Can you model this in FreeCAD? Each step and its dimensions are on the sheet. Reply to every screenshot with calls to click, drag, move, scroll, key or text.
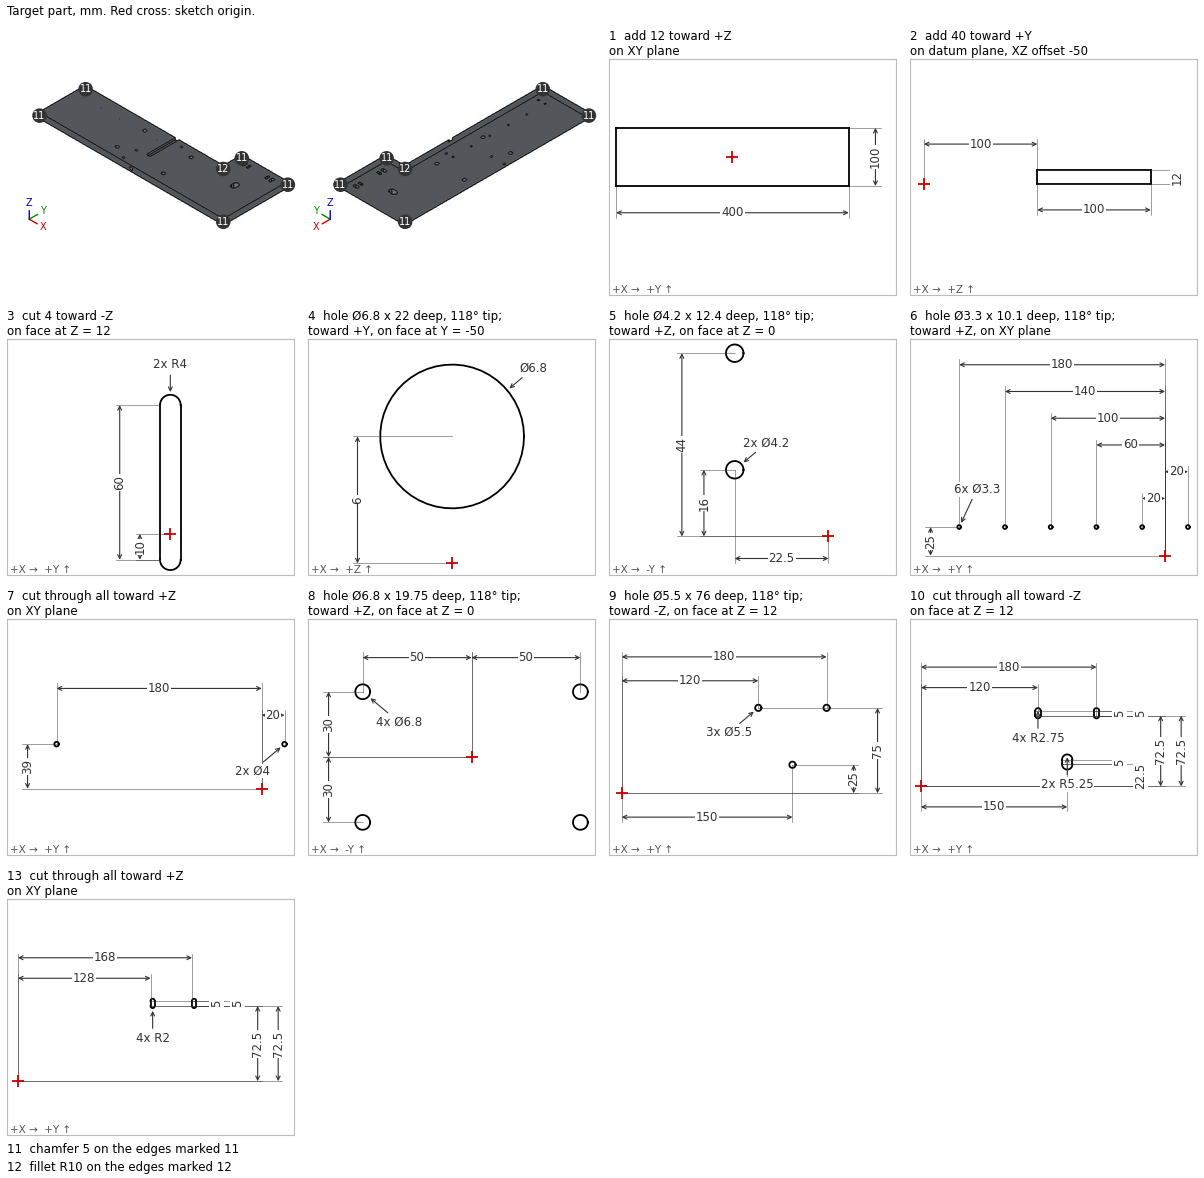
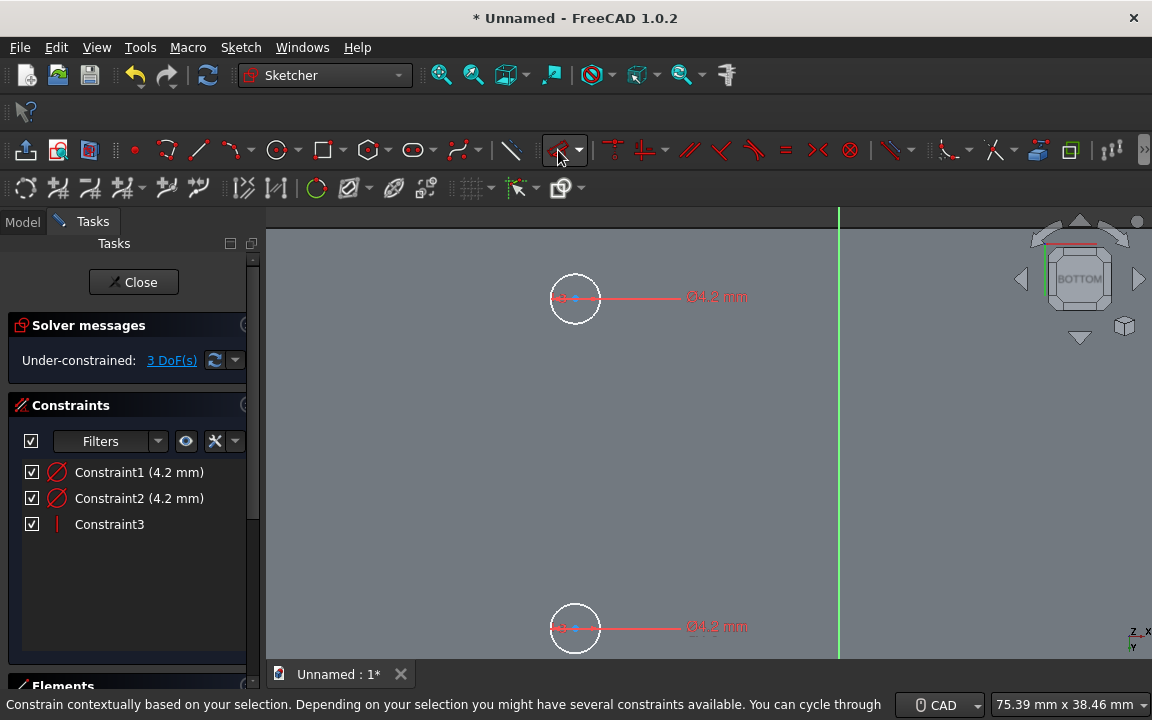
click(575, 629)
click(873, 630)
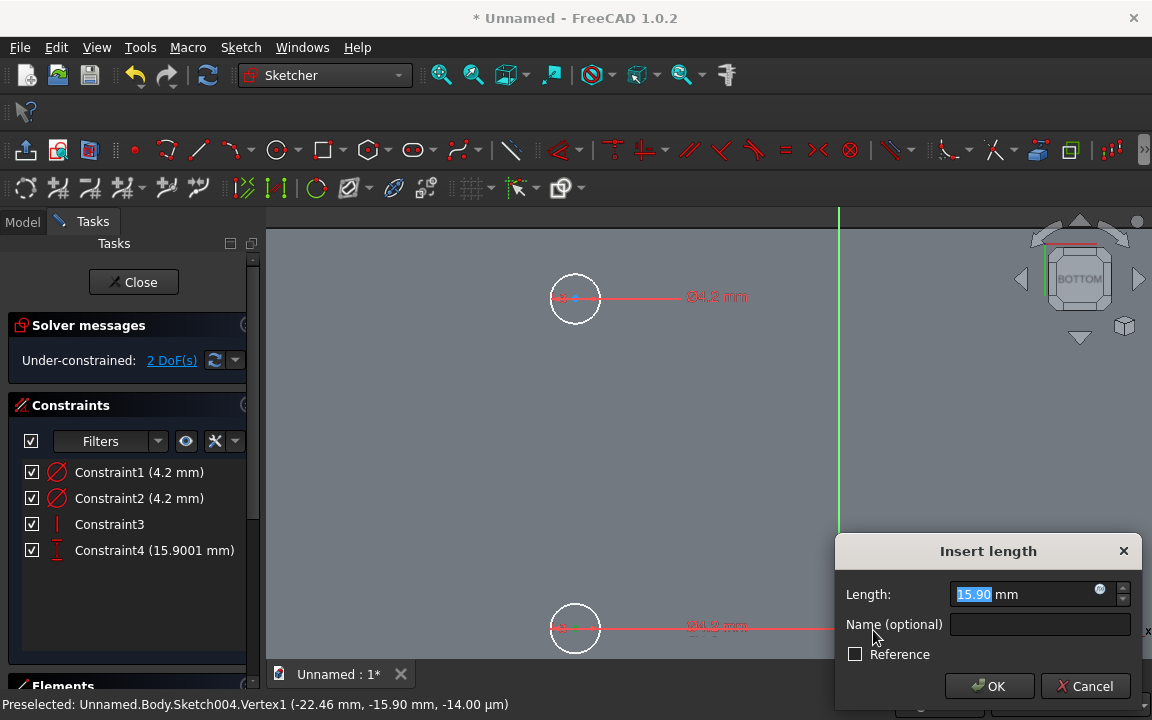
text(16)
key(Return)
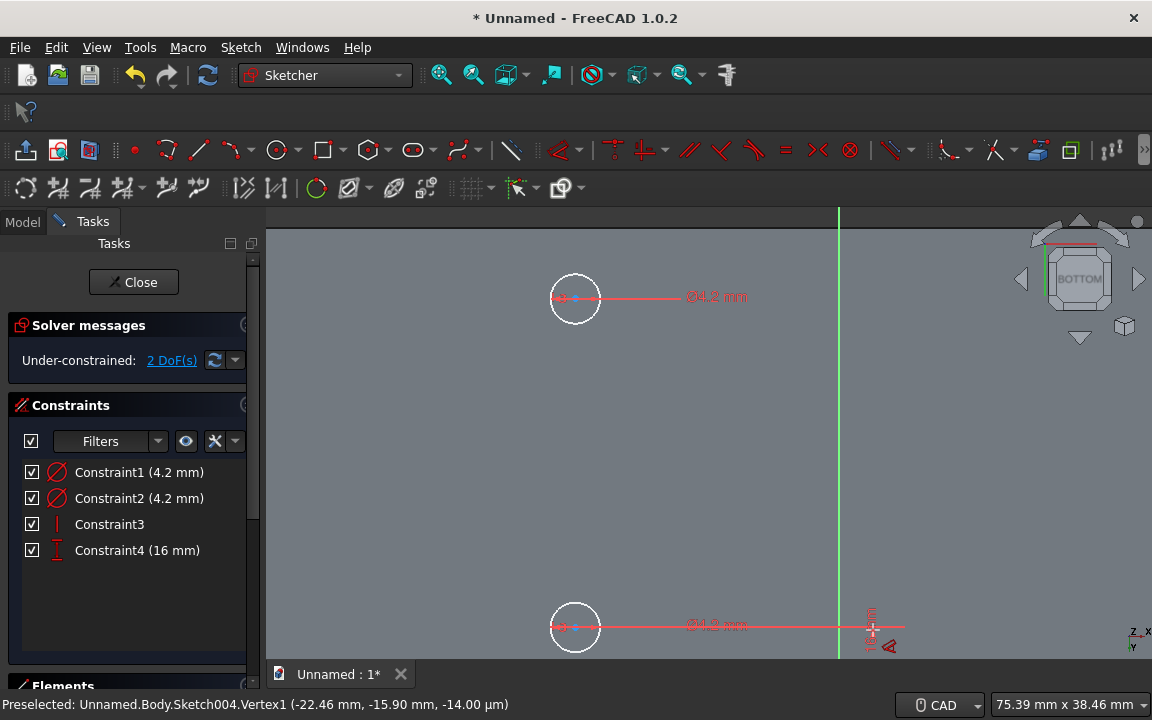
click(575, 299)
click(873, 465)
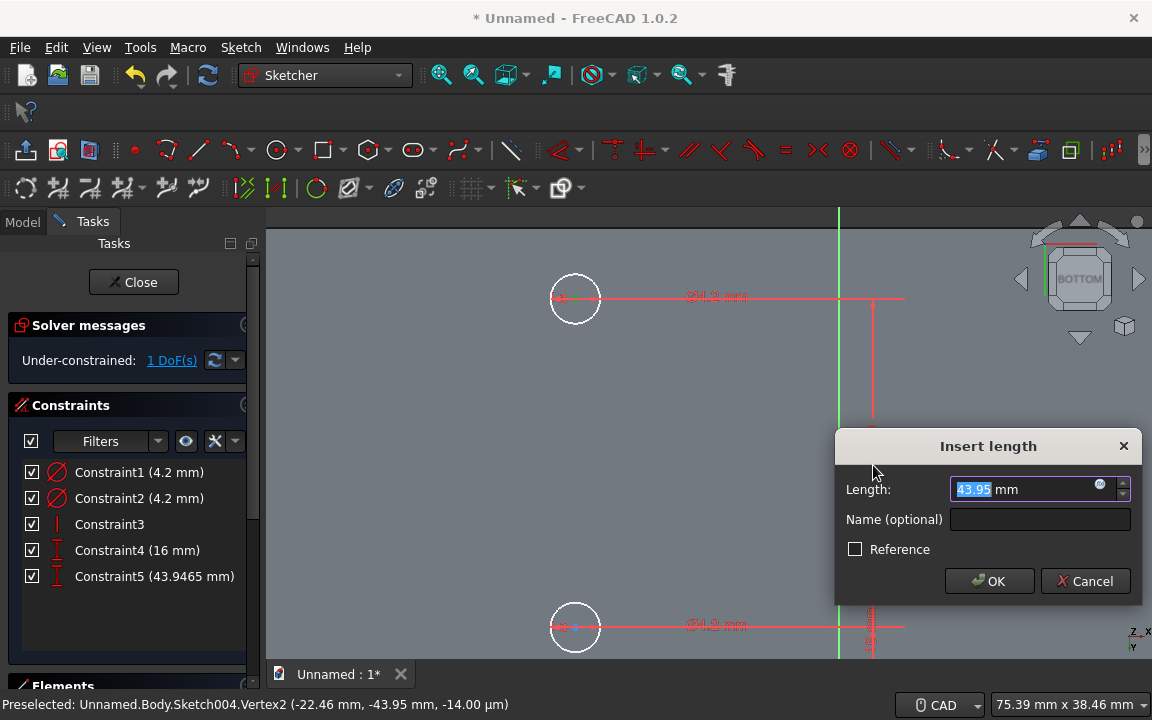
text(44)
key(Return)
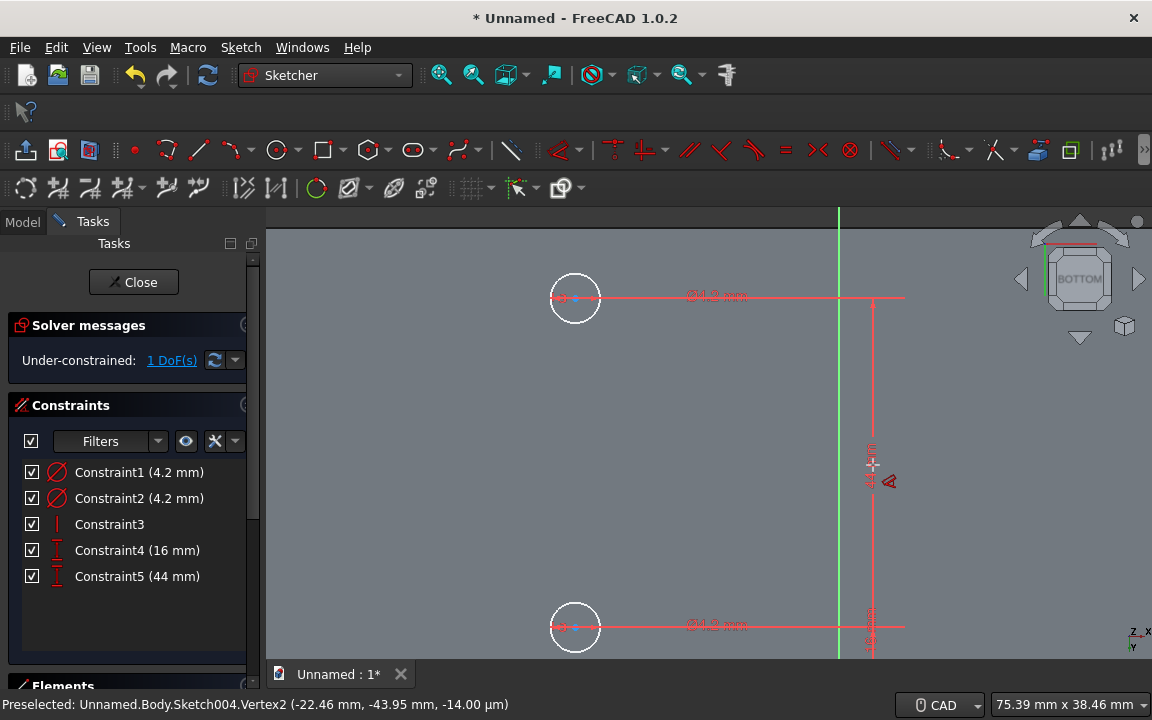
click(575, 627)
click(707, 593)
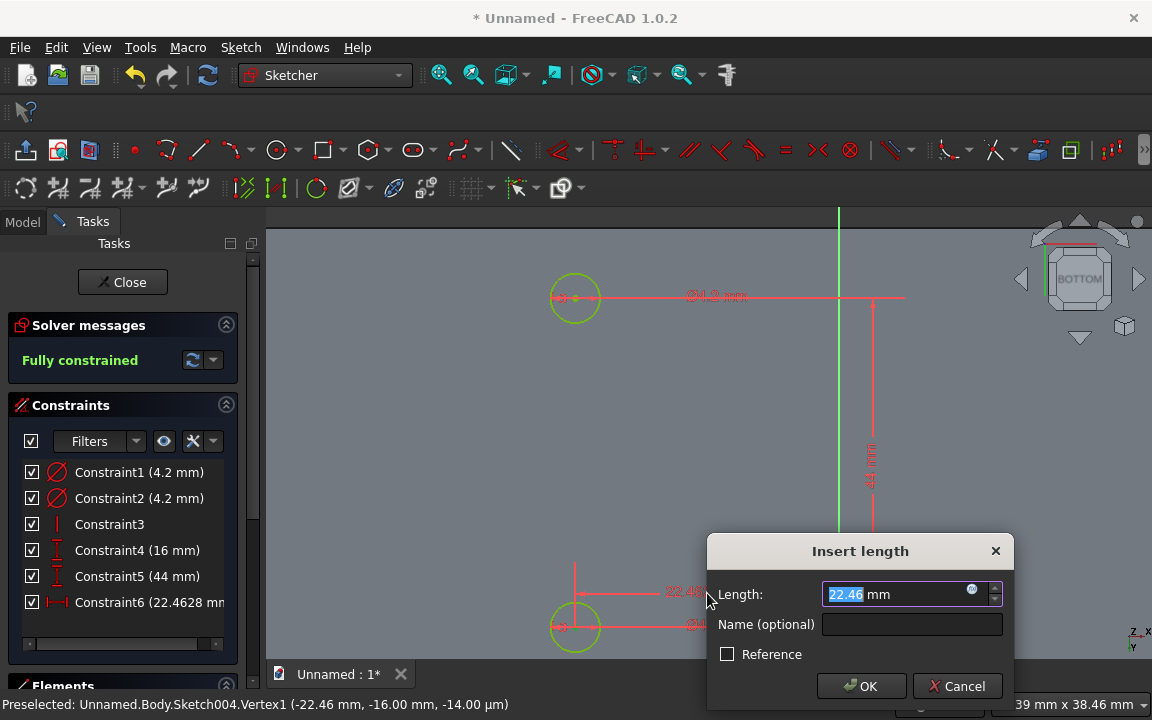
text(22.5)
key(Return)
key(Escape)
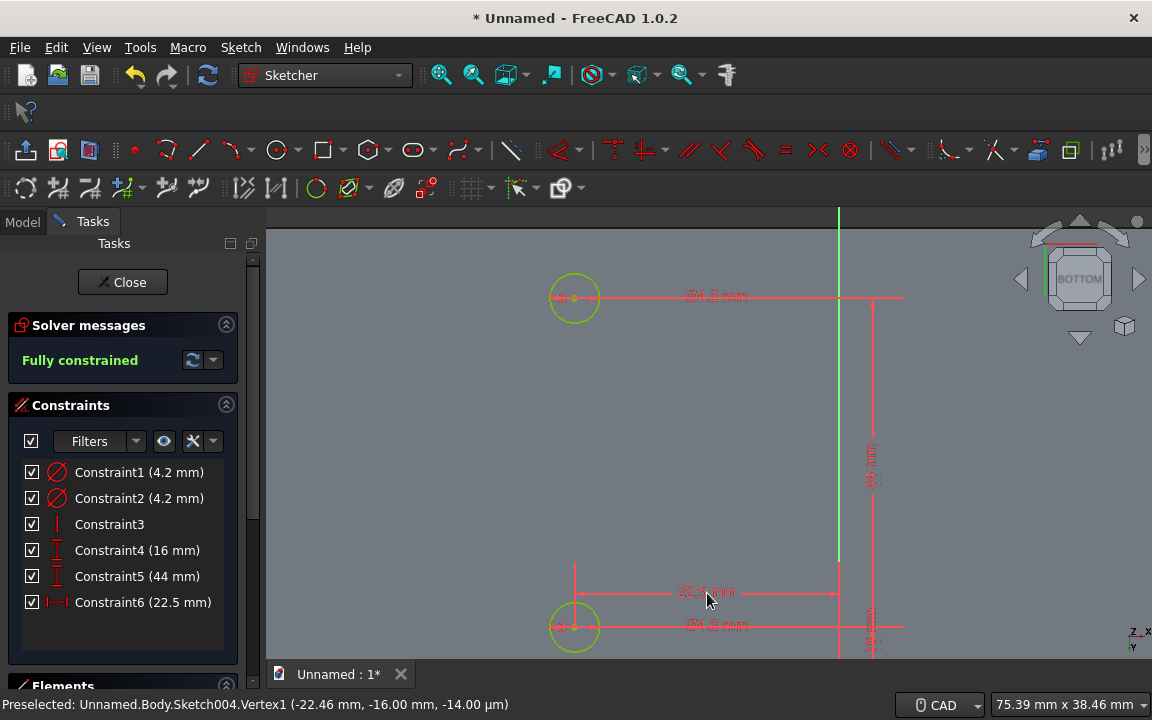
click(123, 282)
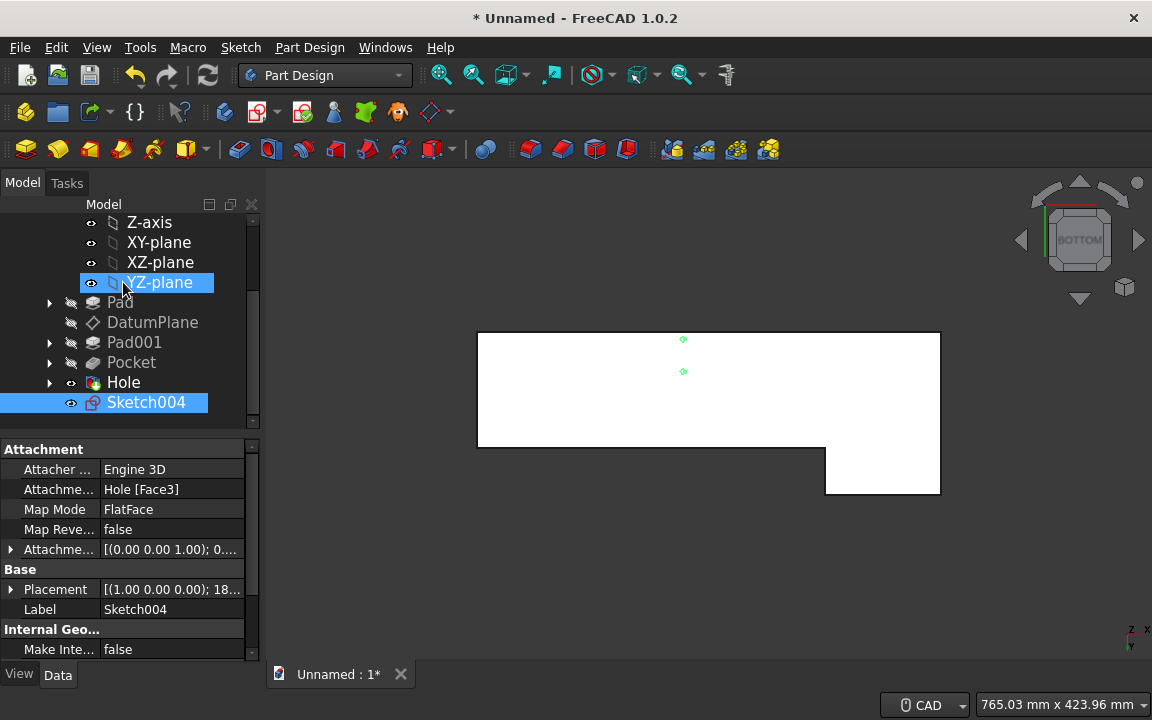
click(272, 150)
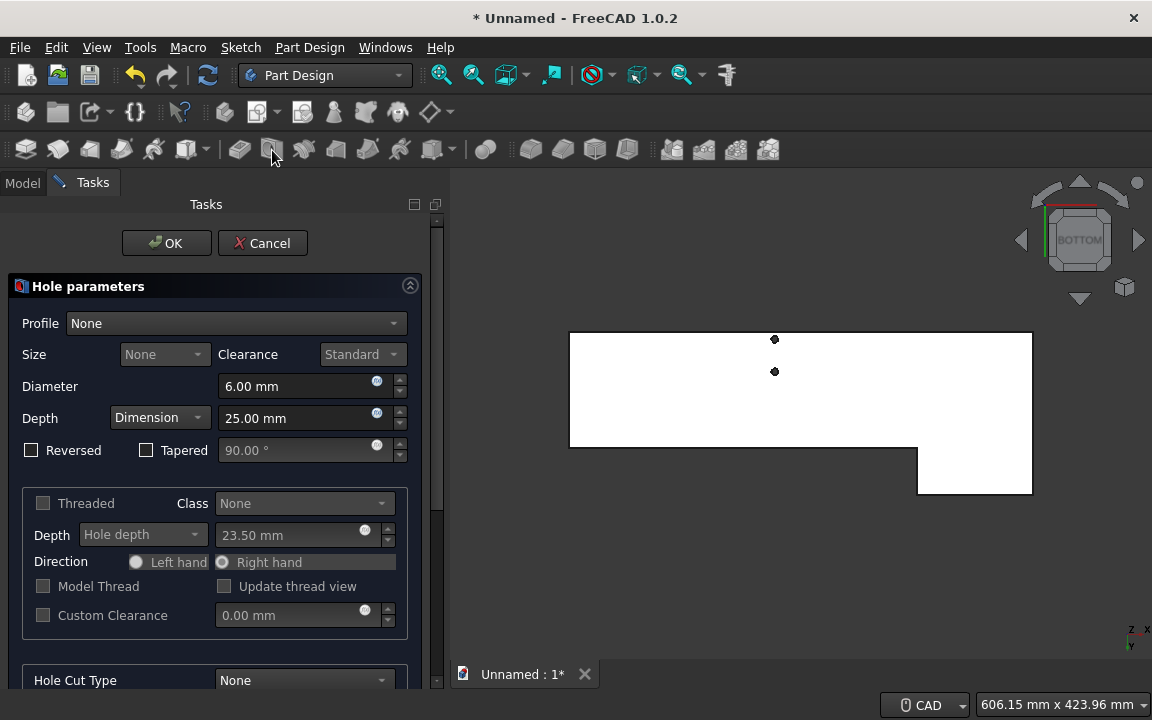
triple_click(305, 386)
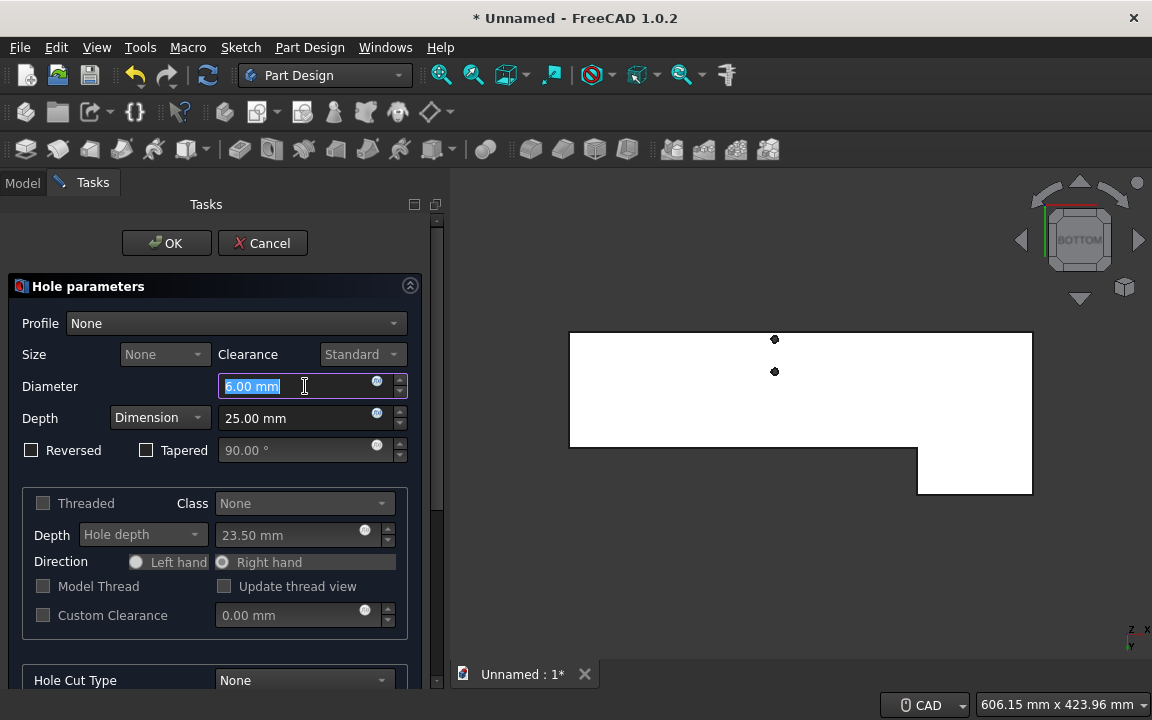
text(4.2)
key(Tab)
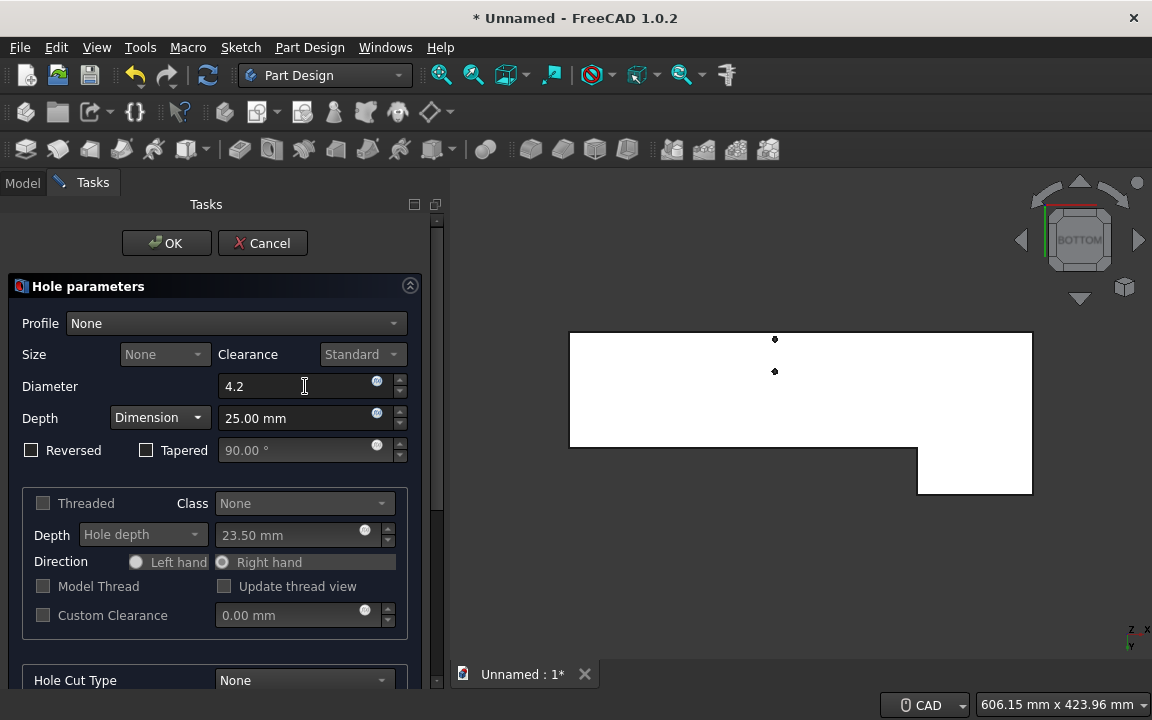
triple_click(305, 418)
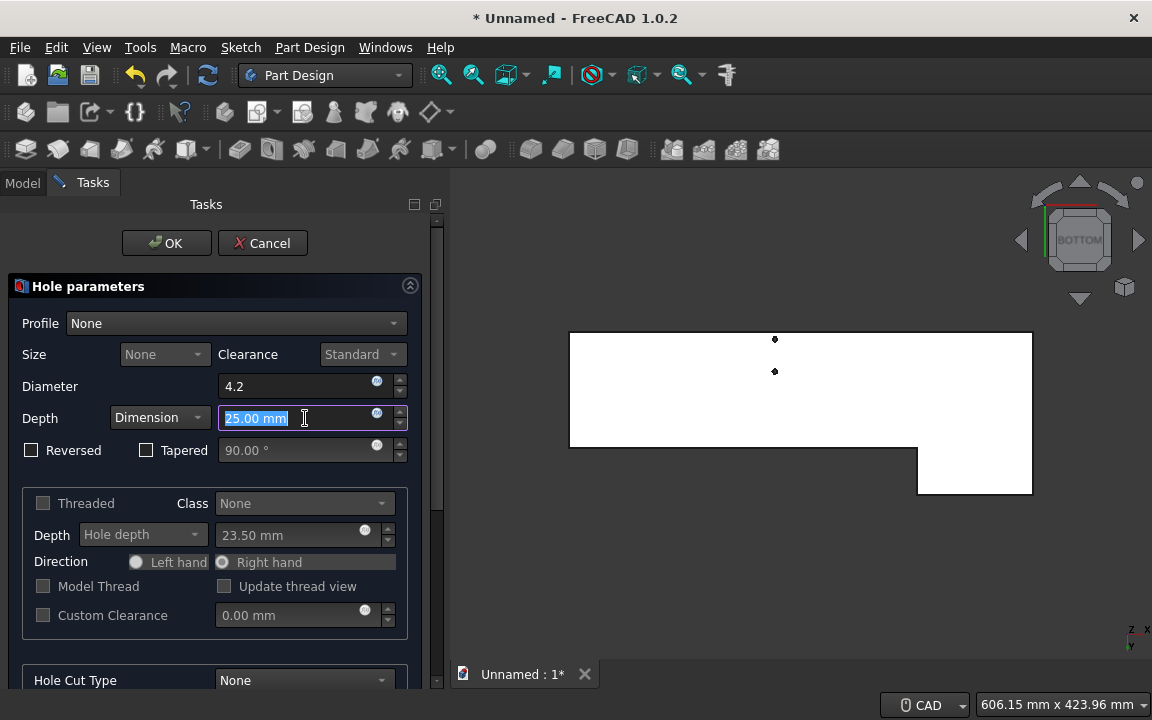
text(12.4)
key(Tab)